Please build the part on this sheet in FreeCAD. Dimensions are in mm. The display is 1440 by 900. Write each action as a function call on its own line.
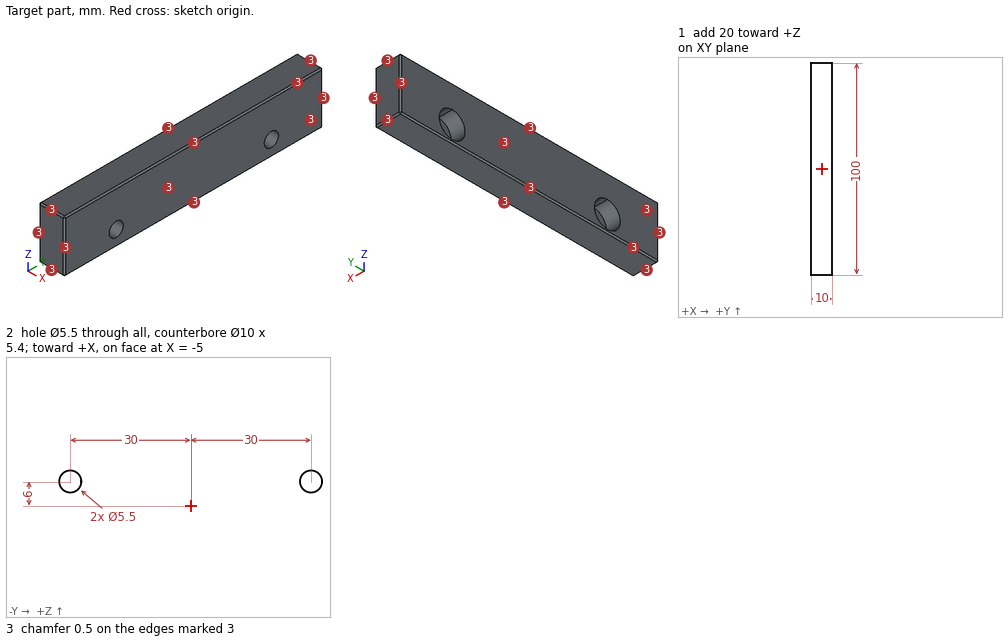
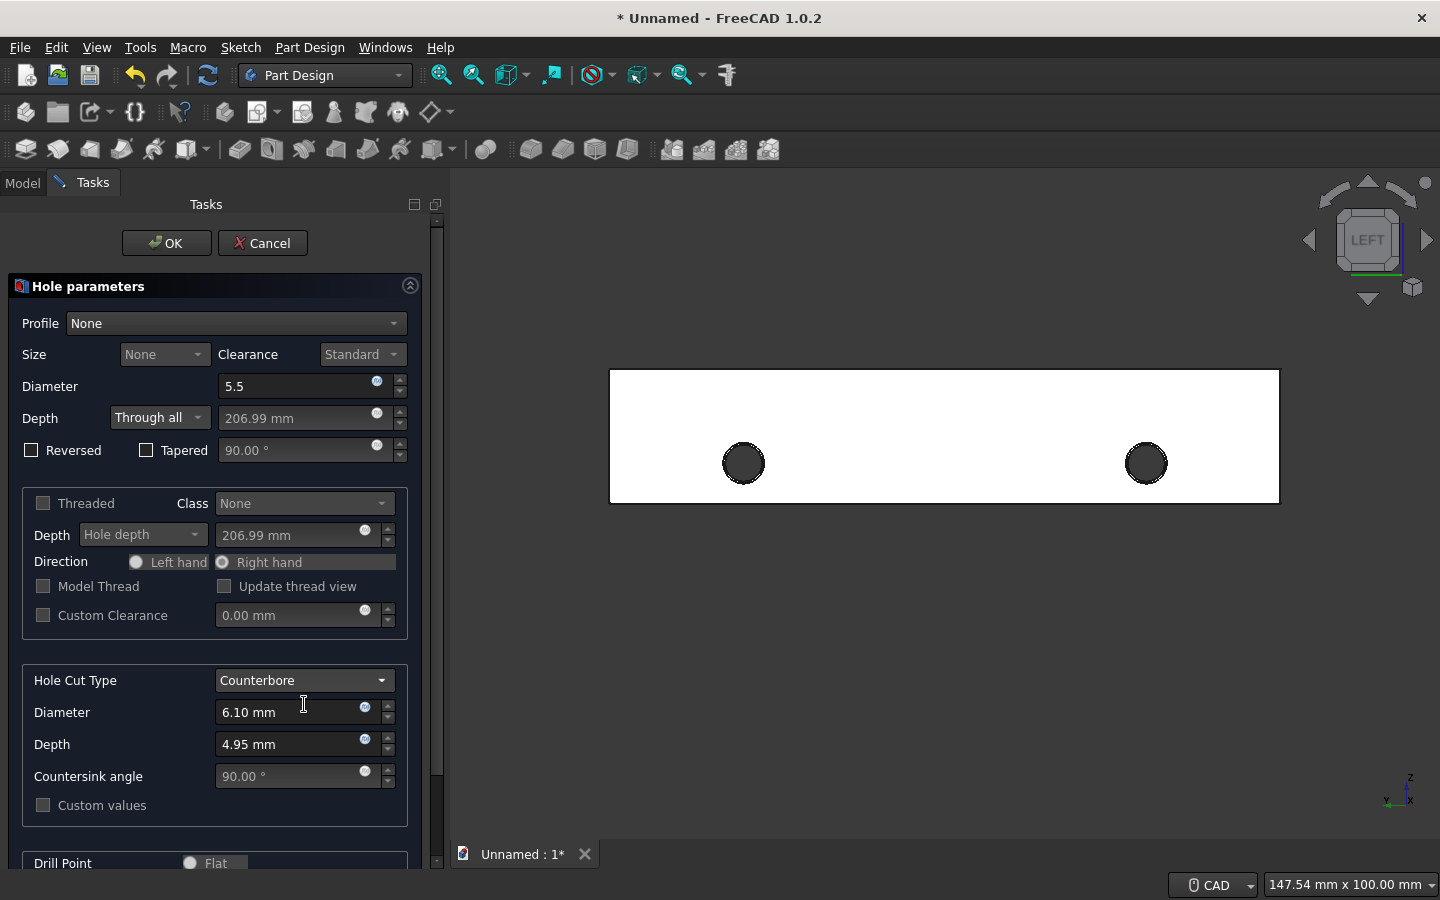
triple_click(298, 712)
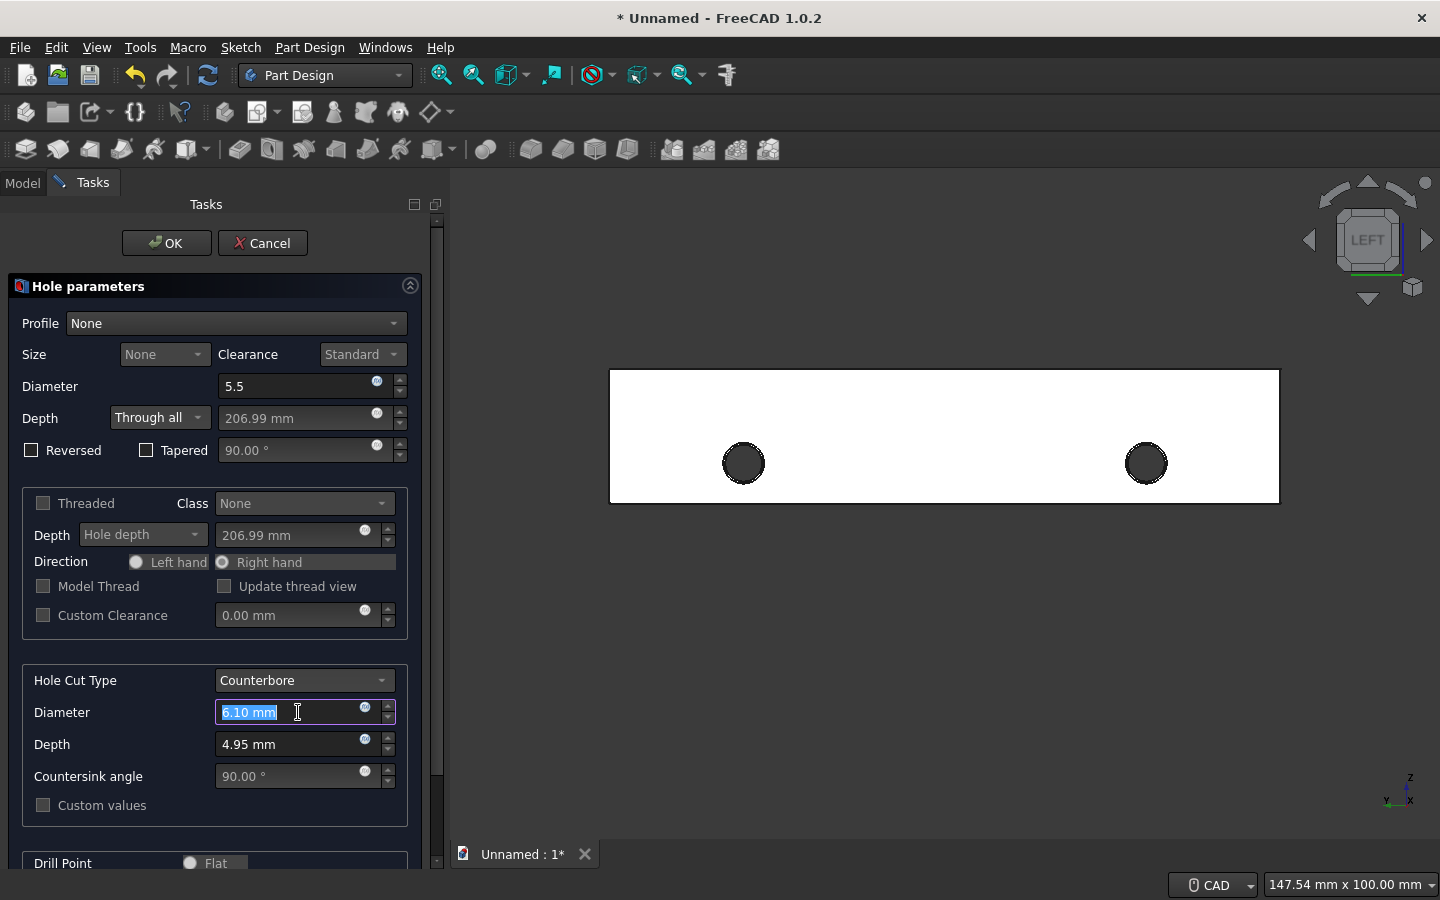
text(10)
key(Tab)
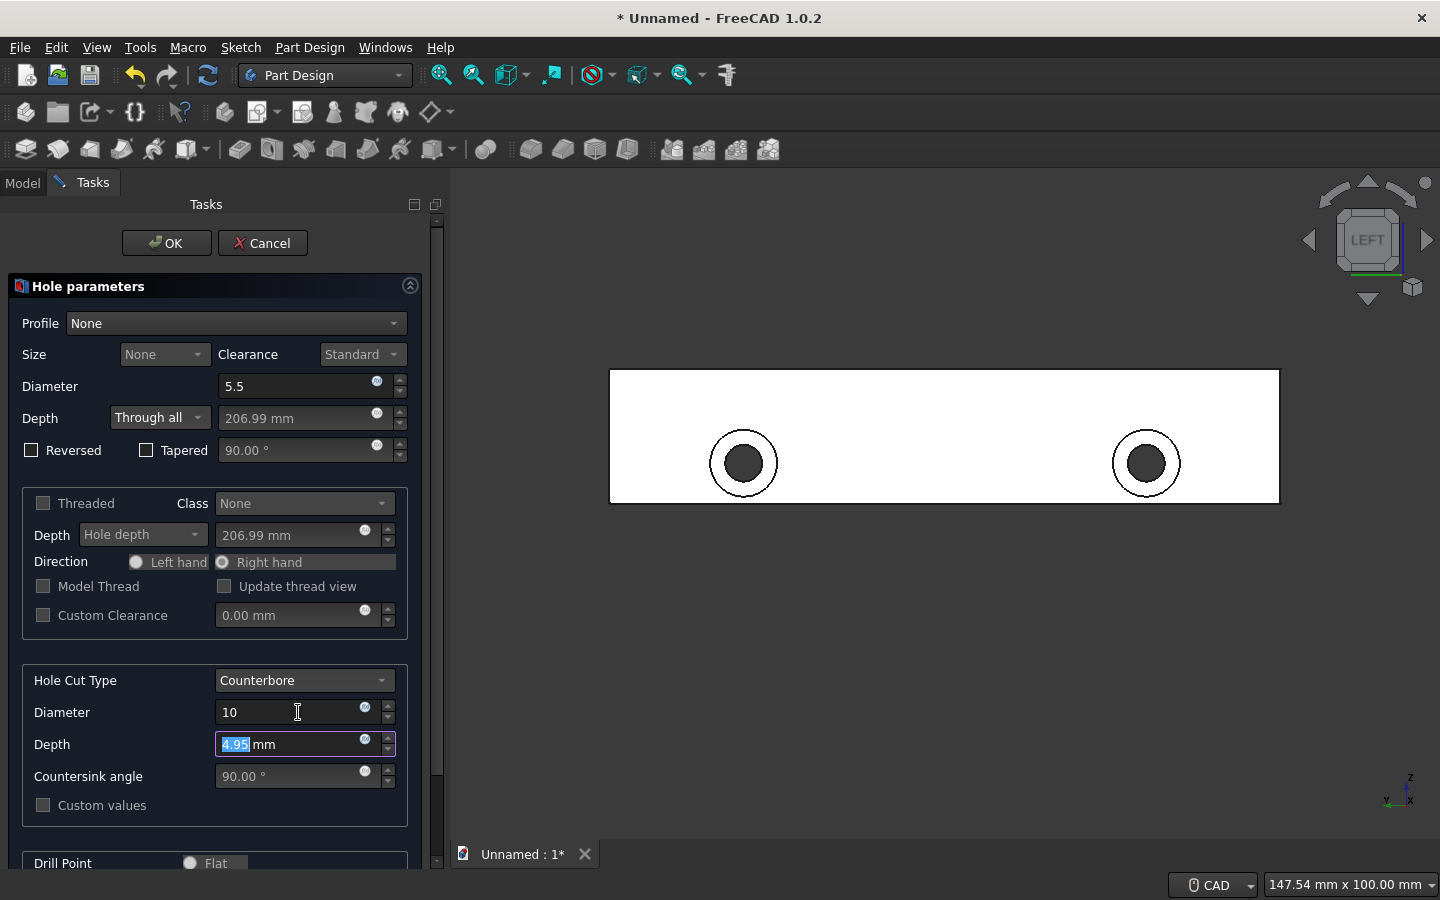
text(5.4)
key(Tab)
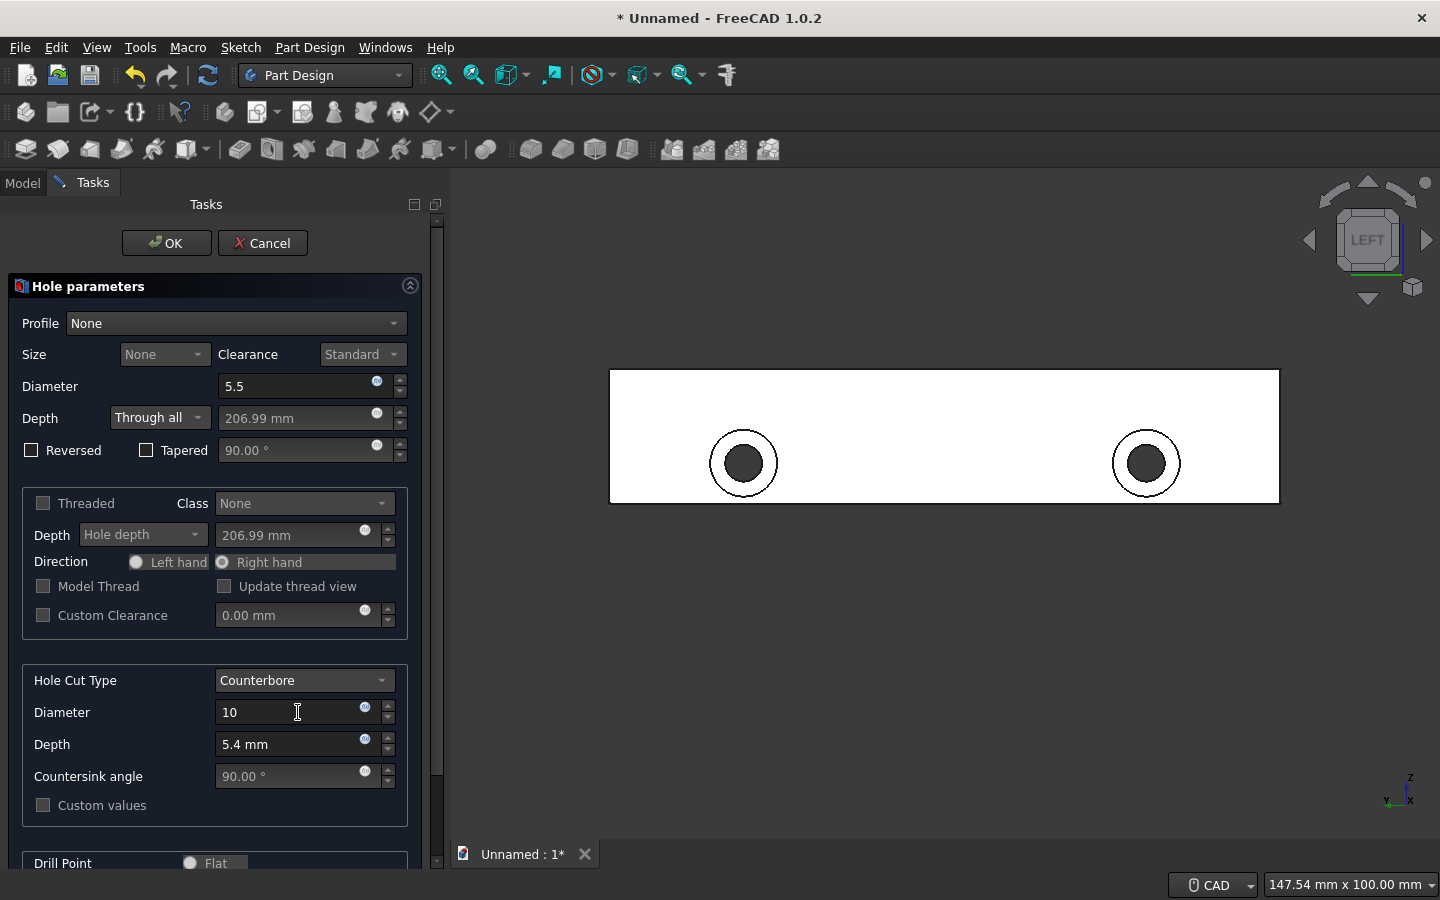
click(167, 243)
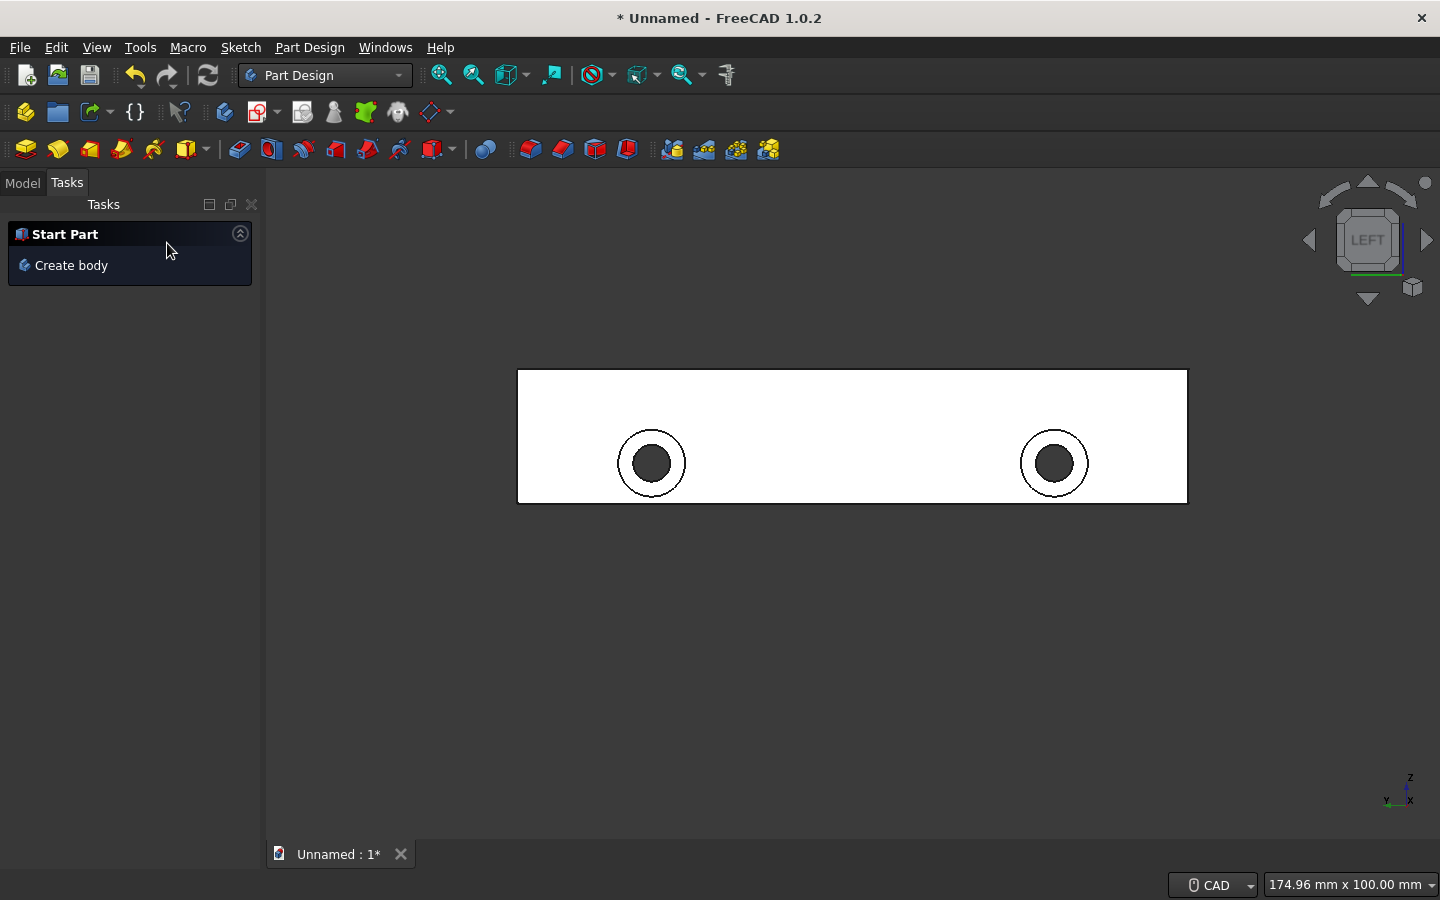
click(1189, 435)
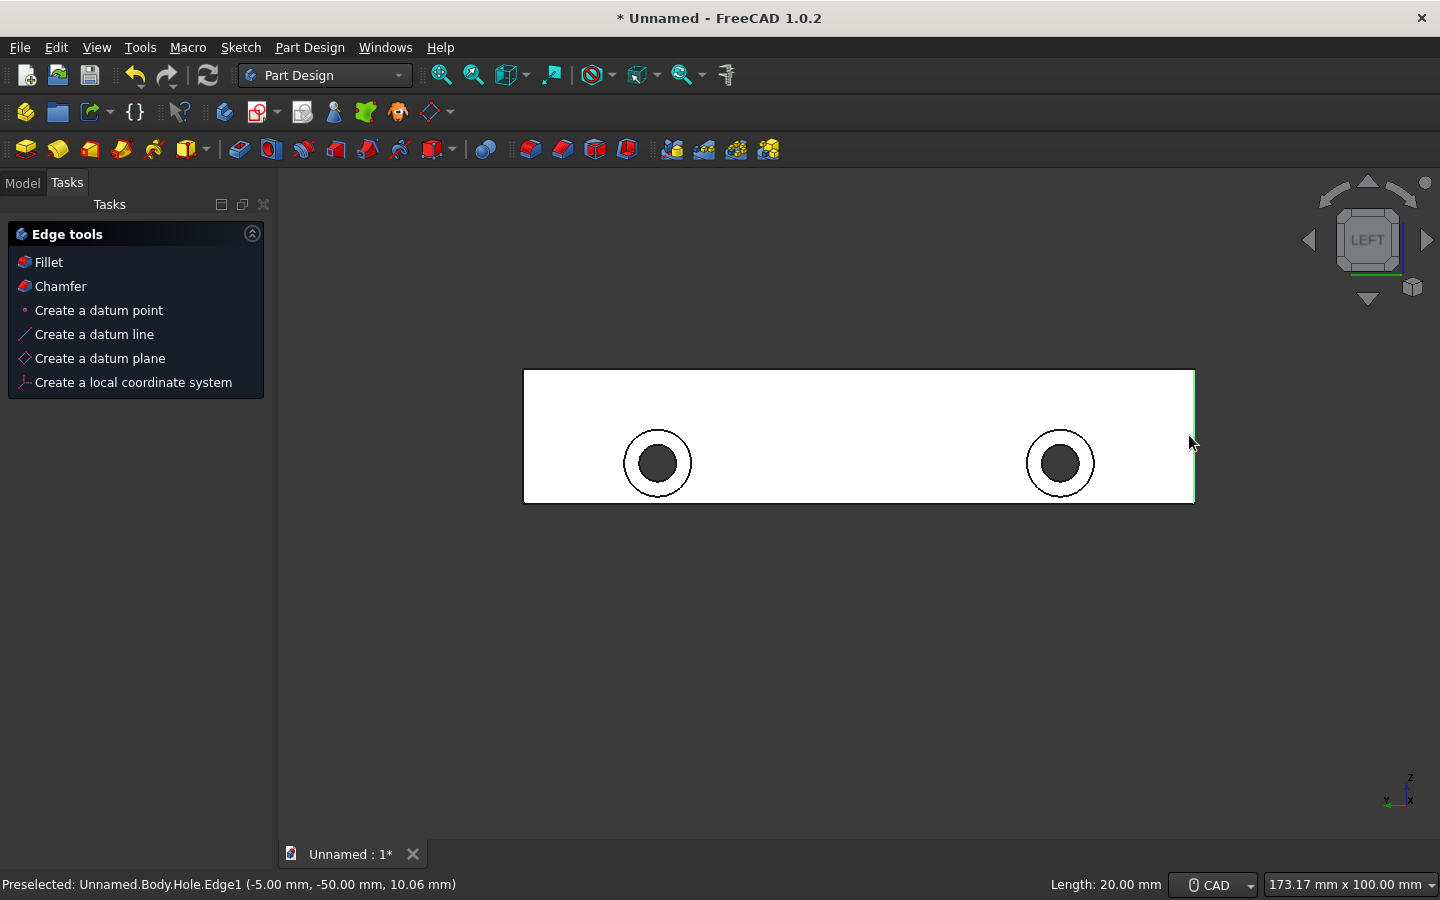
click(523, 435, ctrl)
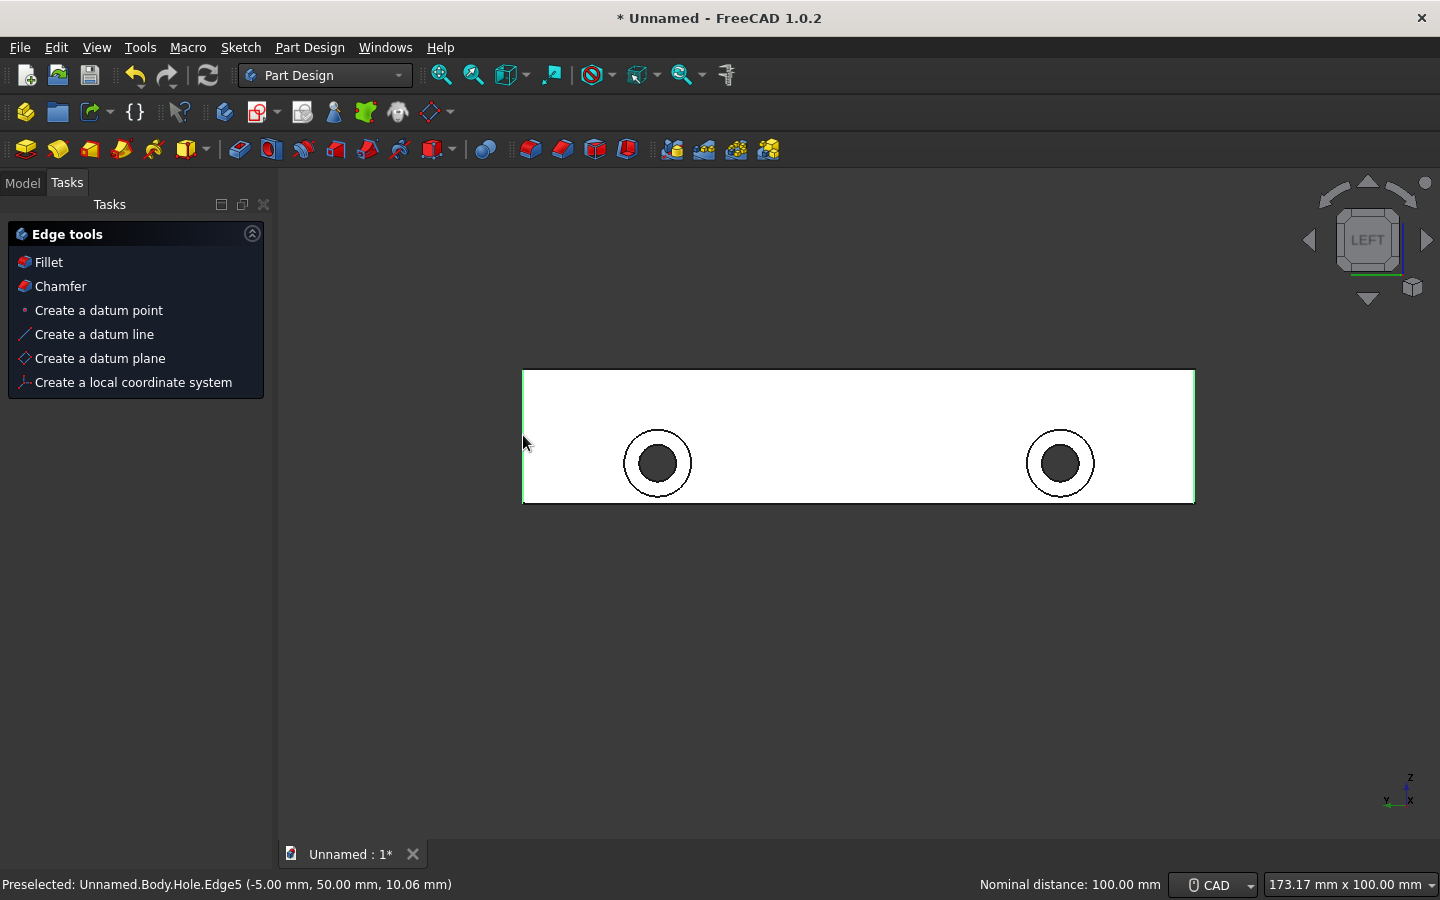
key(0)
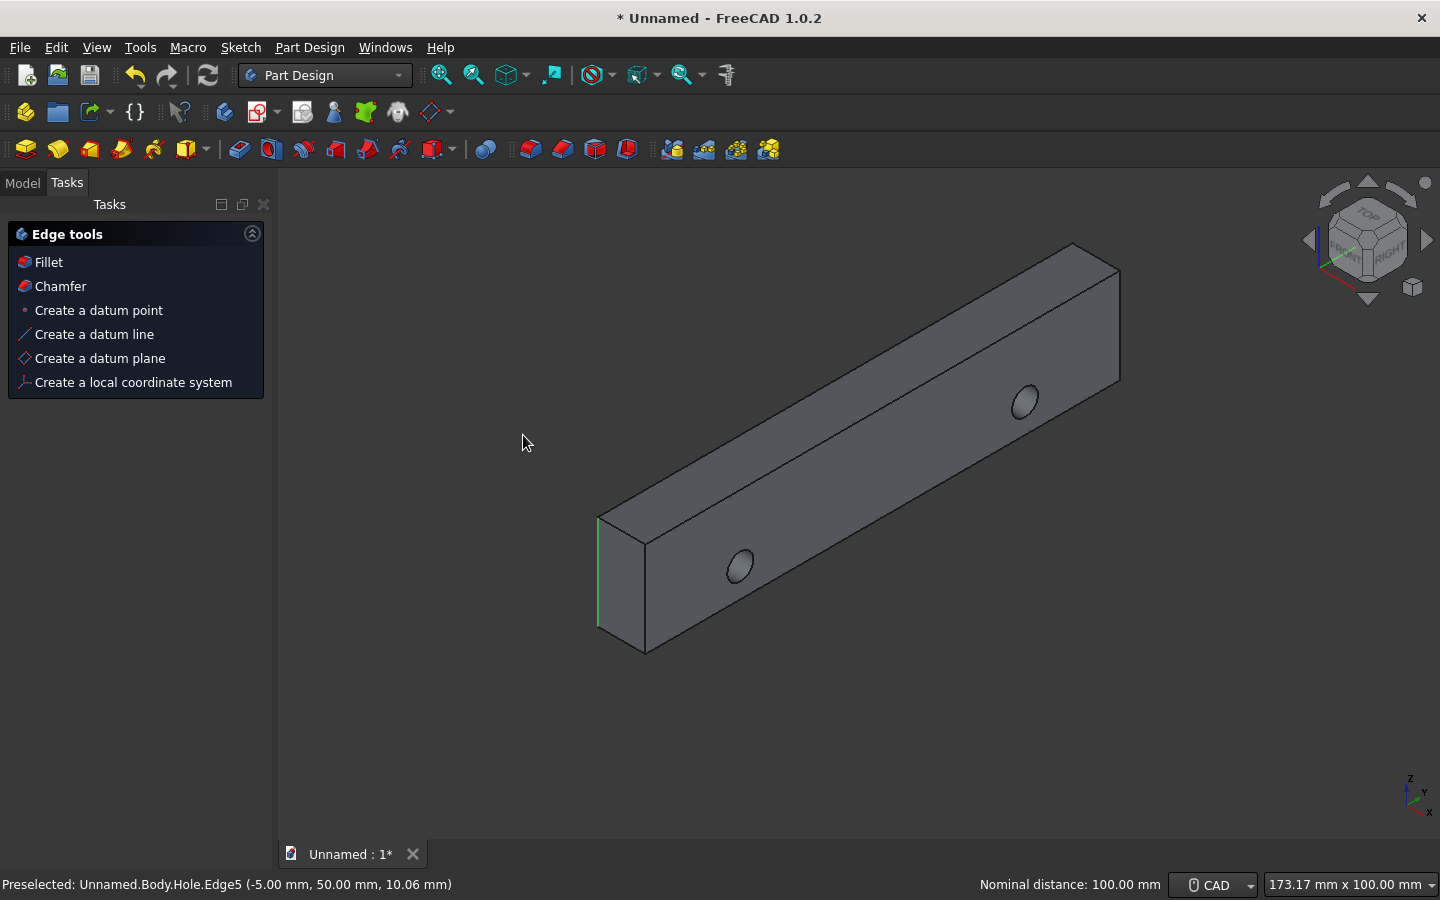
click(1062, 276, ctrl)